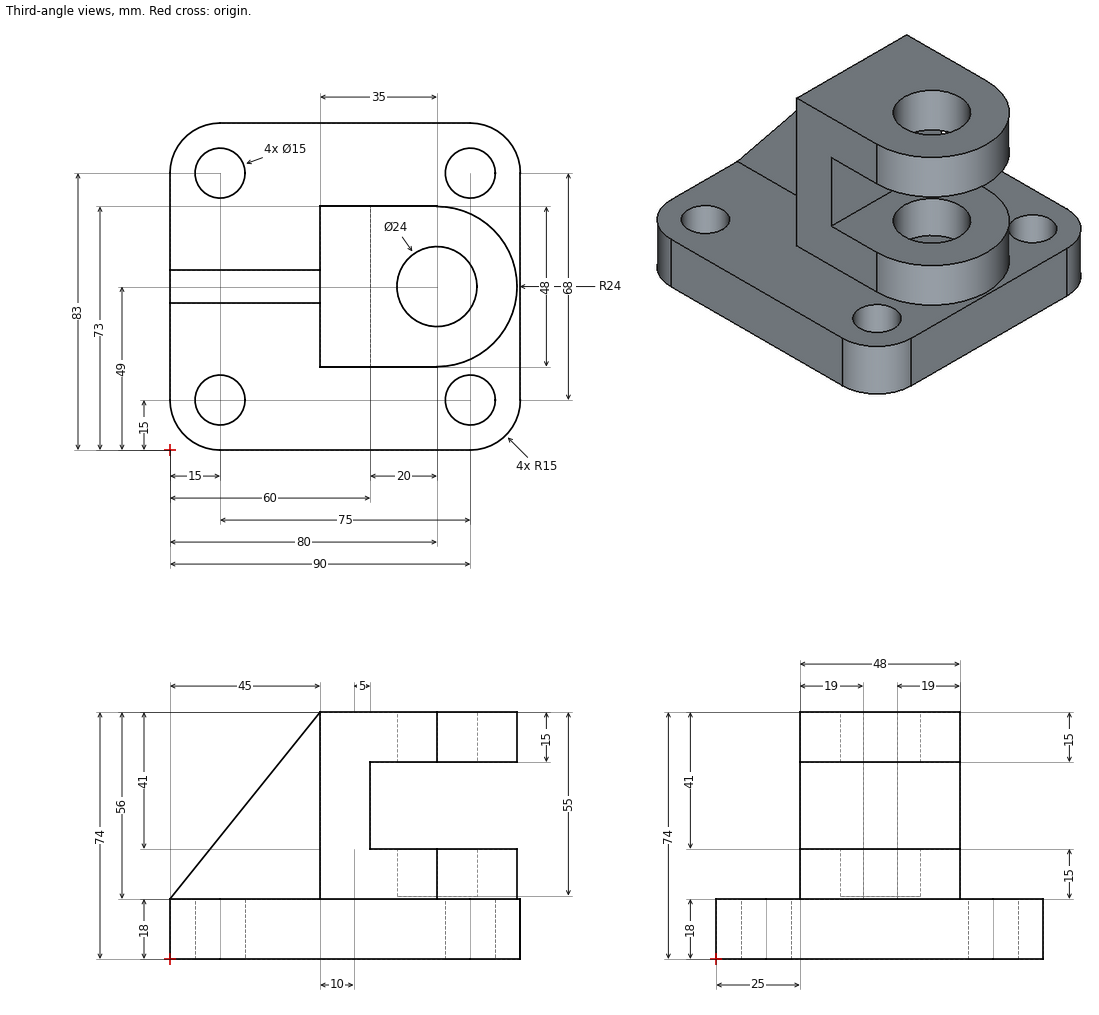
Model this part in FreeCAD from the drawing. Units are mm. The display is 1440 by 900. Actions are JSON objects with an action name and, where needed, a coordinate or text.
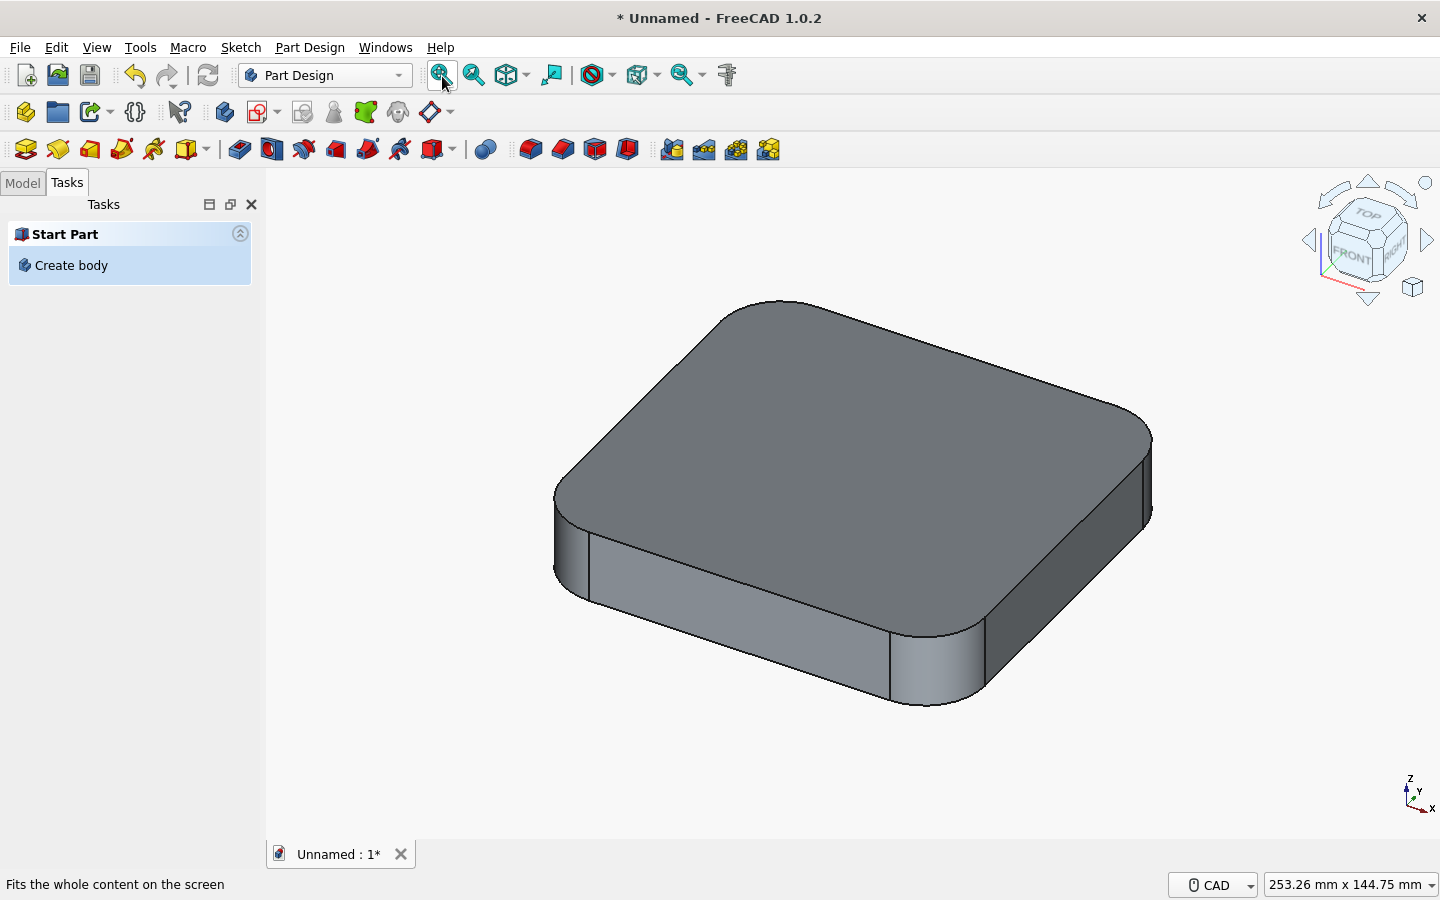
{"action": "left_click", "coordinate": [853, 468]}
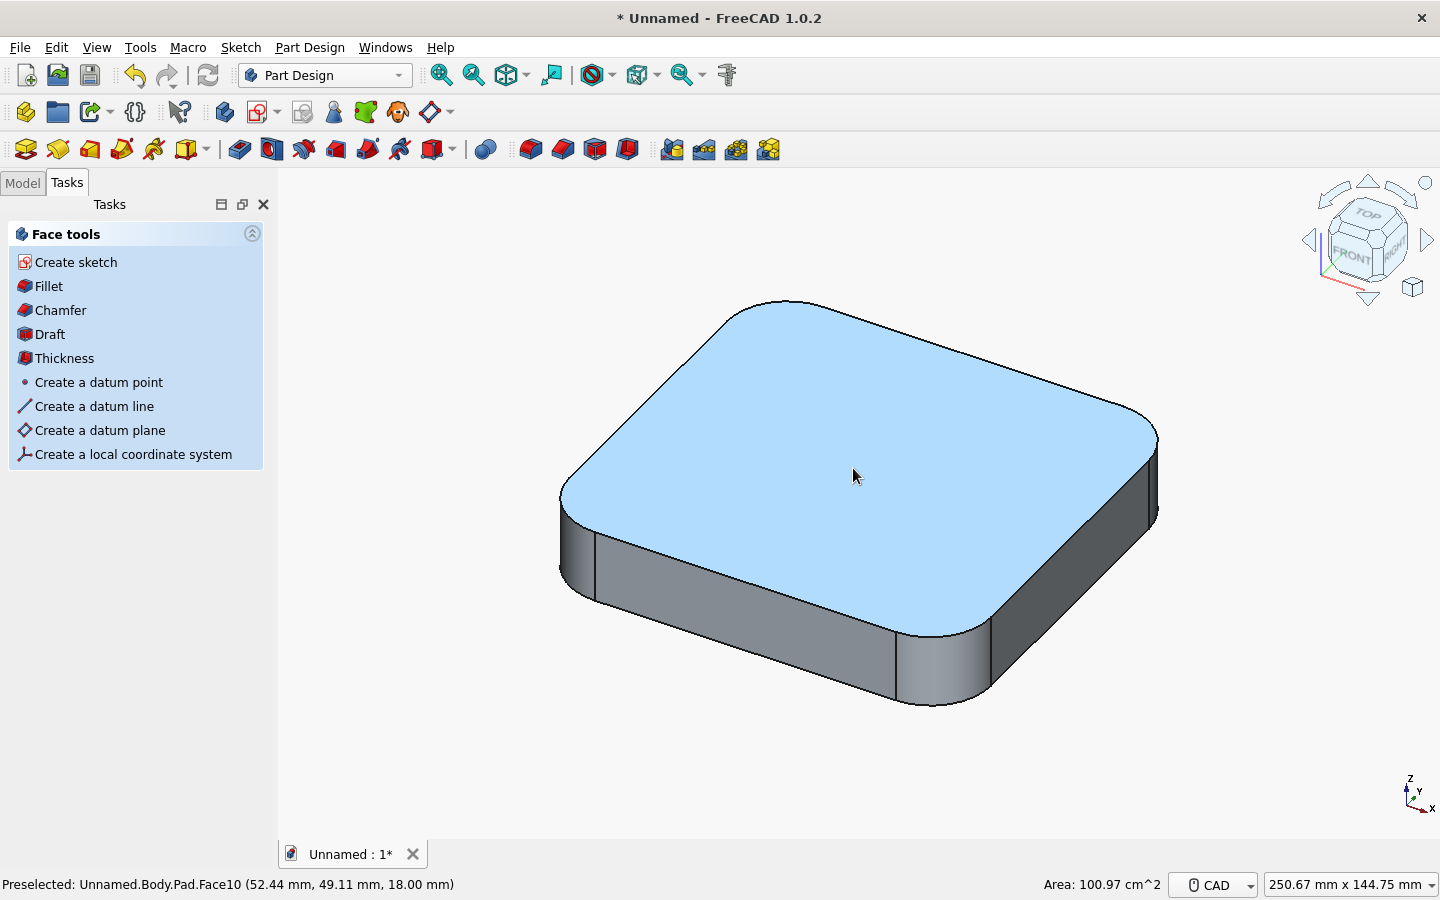
{"action": "left_click", "coordinate": [258, 112]}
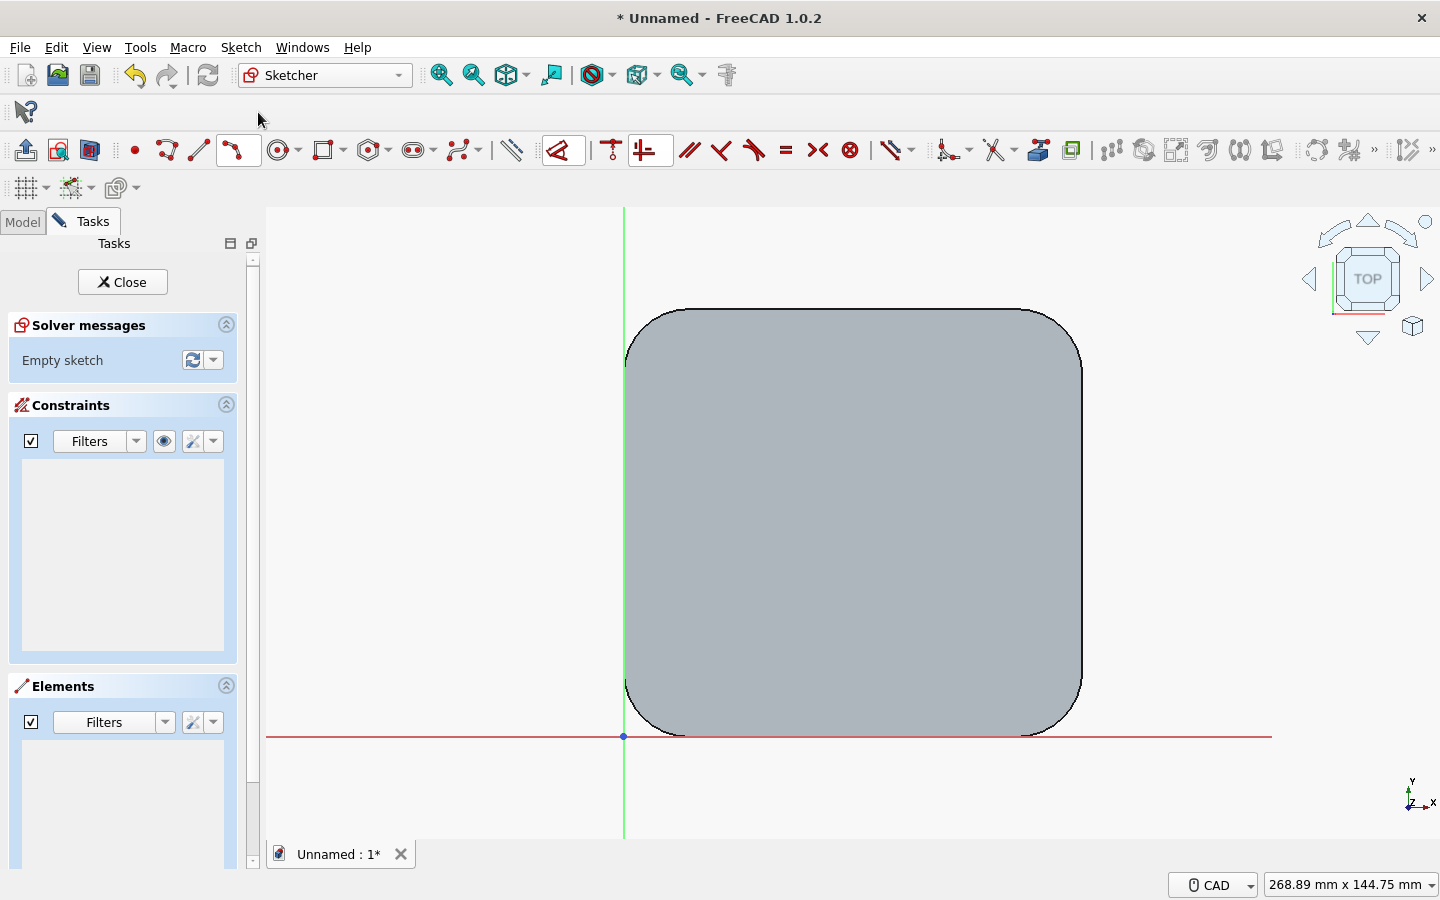
{"action": "left_click", "coordinate": [278, 150]}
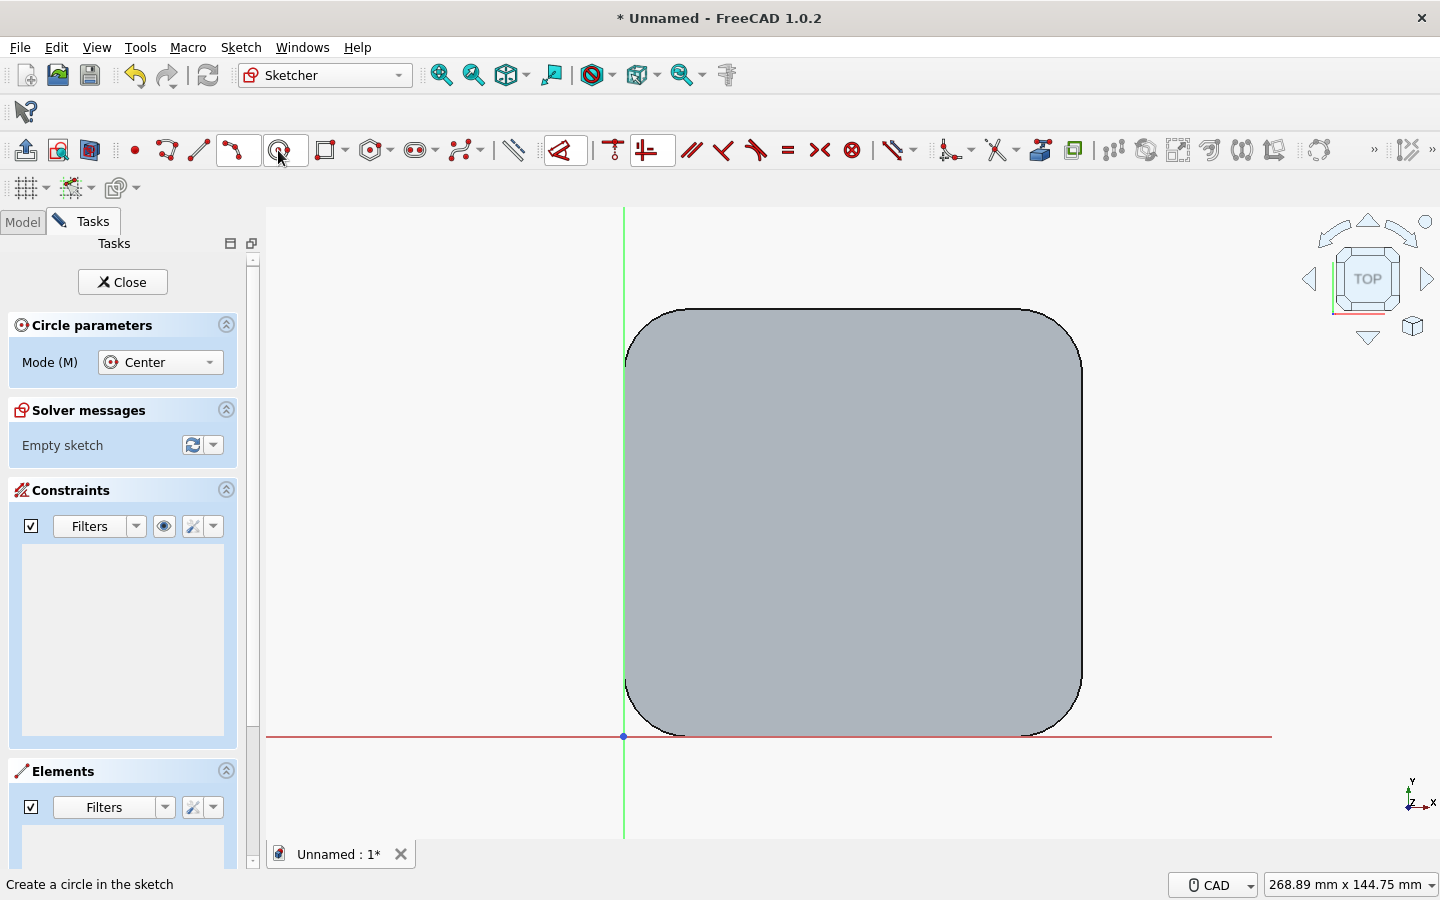
{"action": "left_click", "coordinate": [689, 375]}
{"action": "left_click", "coordinate": [712, 351]}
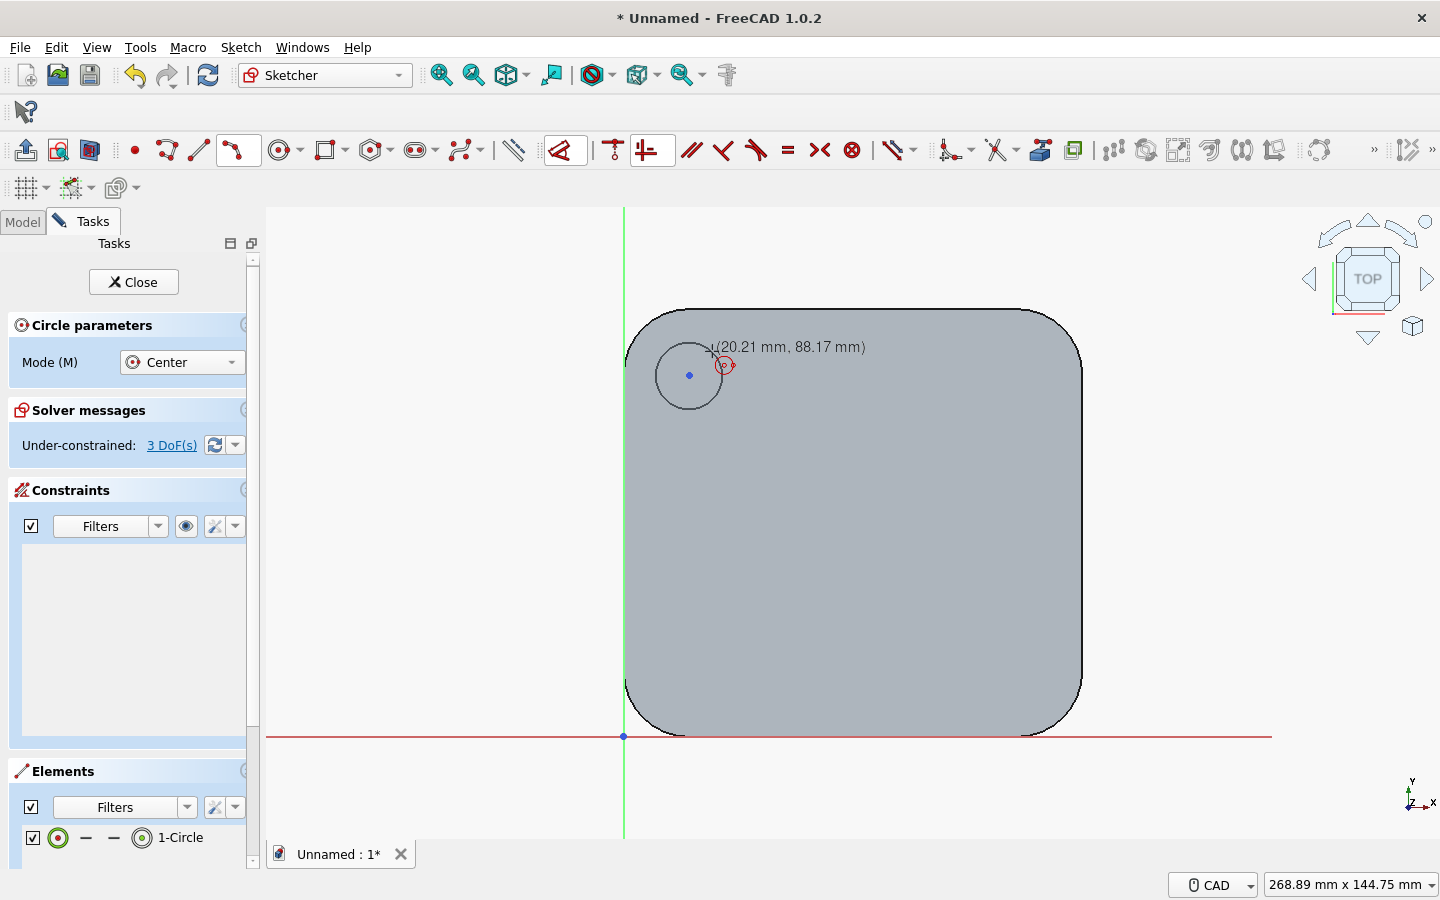
{"action": "left_click", "coordinate": [1017, 375]}
{"action": "left_click", "coordinate": [1040, 351]}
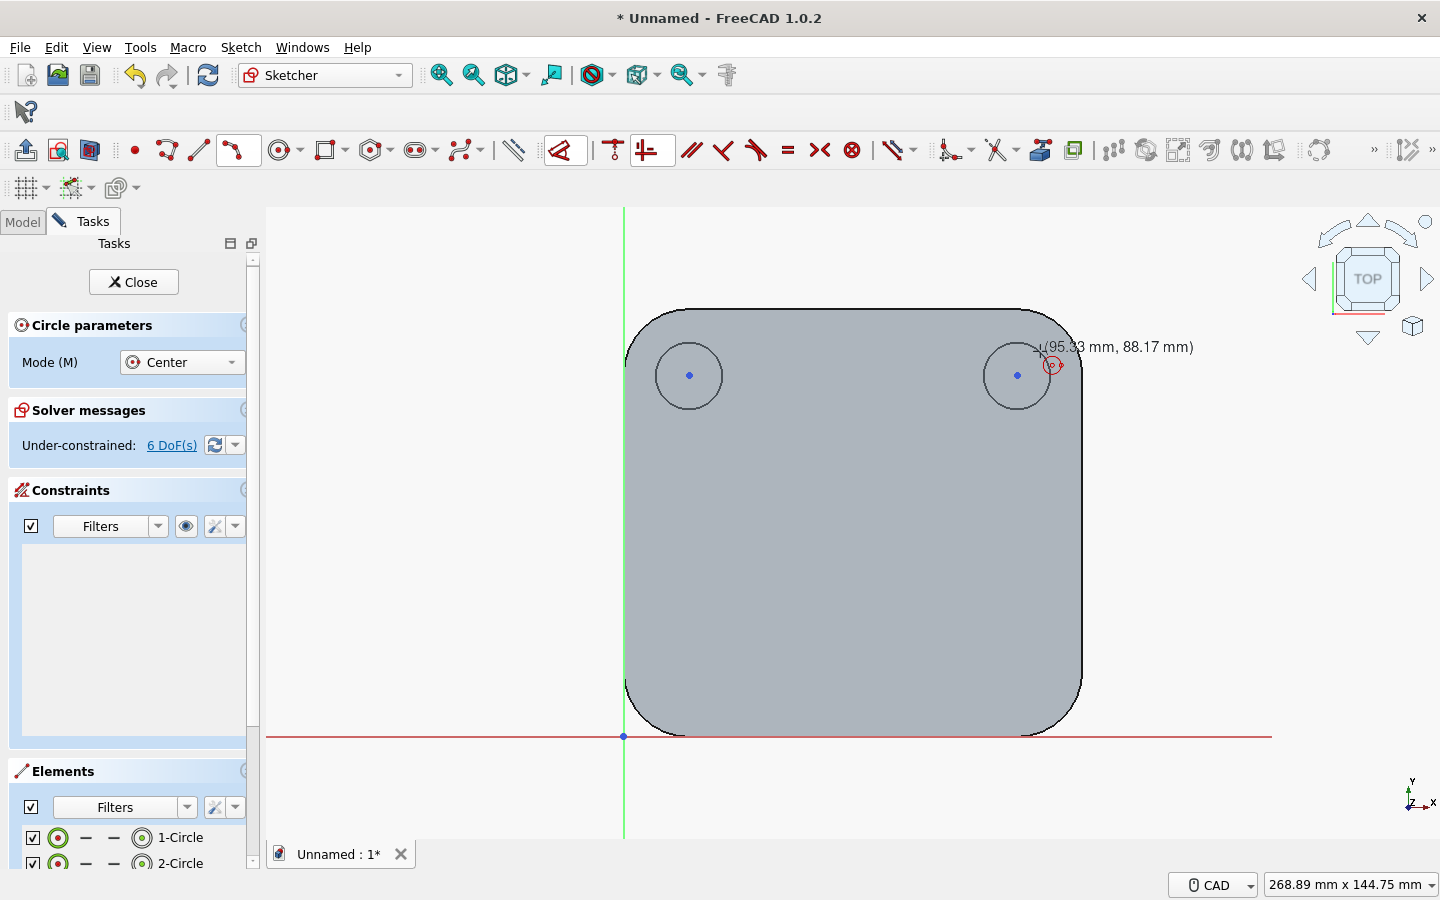
{"action": "left_click", "coordinate": [1017, 671]}
{"action": "left_click", "coordinate": [1040, 648]}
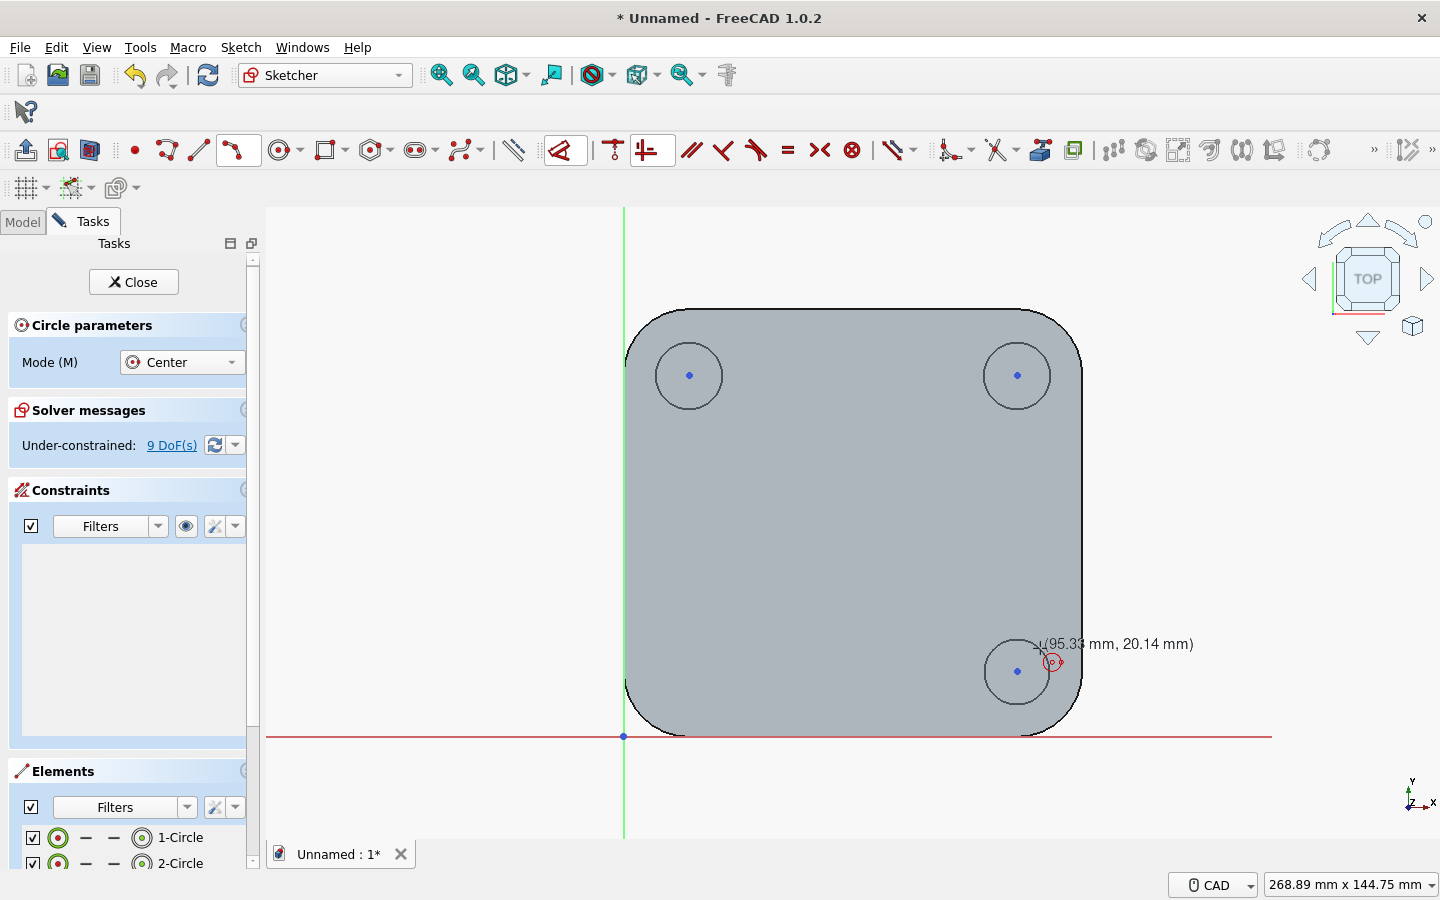
{"action": "left_click", "coordinate": [689, 671]}
{"action": "left_click", "coordinate": [712, 648]}
{"action": "key", "text": "Escape"}